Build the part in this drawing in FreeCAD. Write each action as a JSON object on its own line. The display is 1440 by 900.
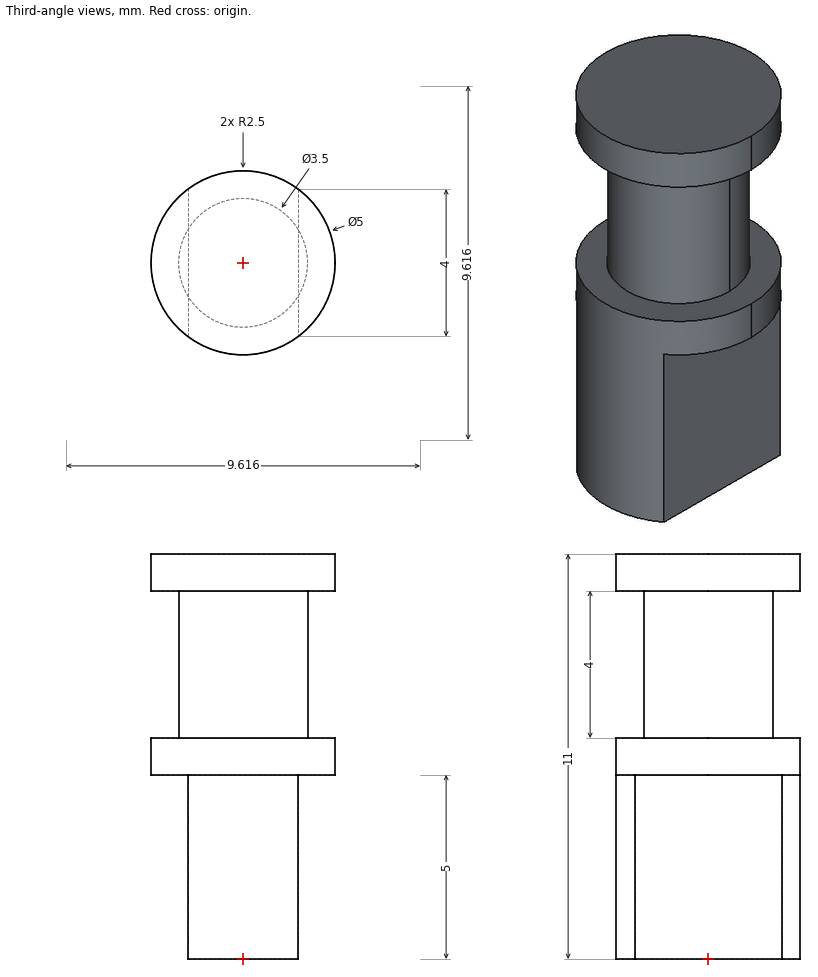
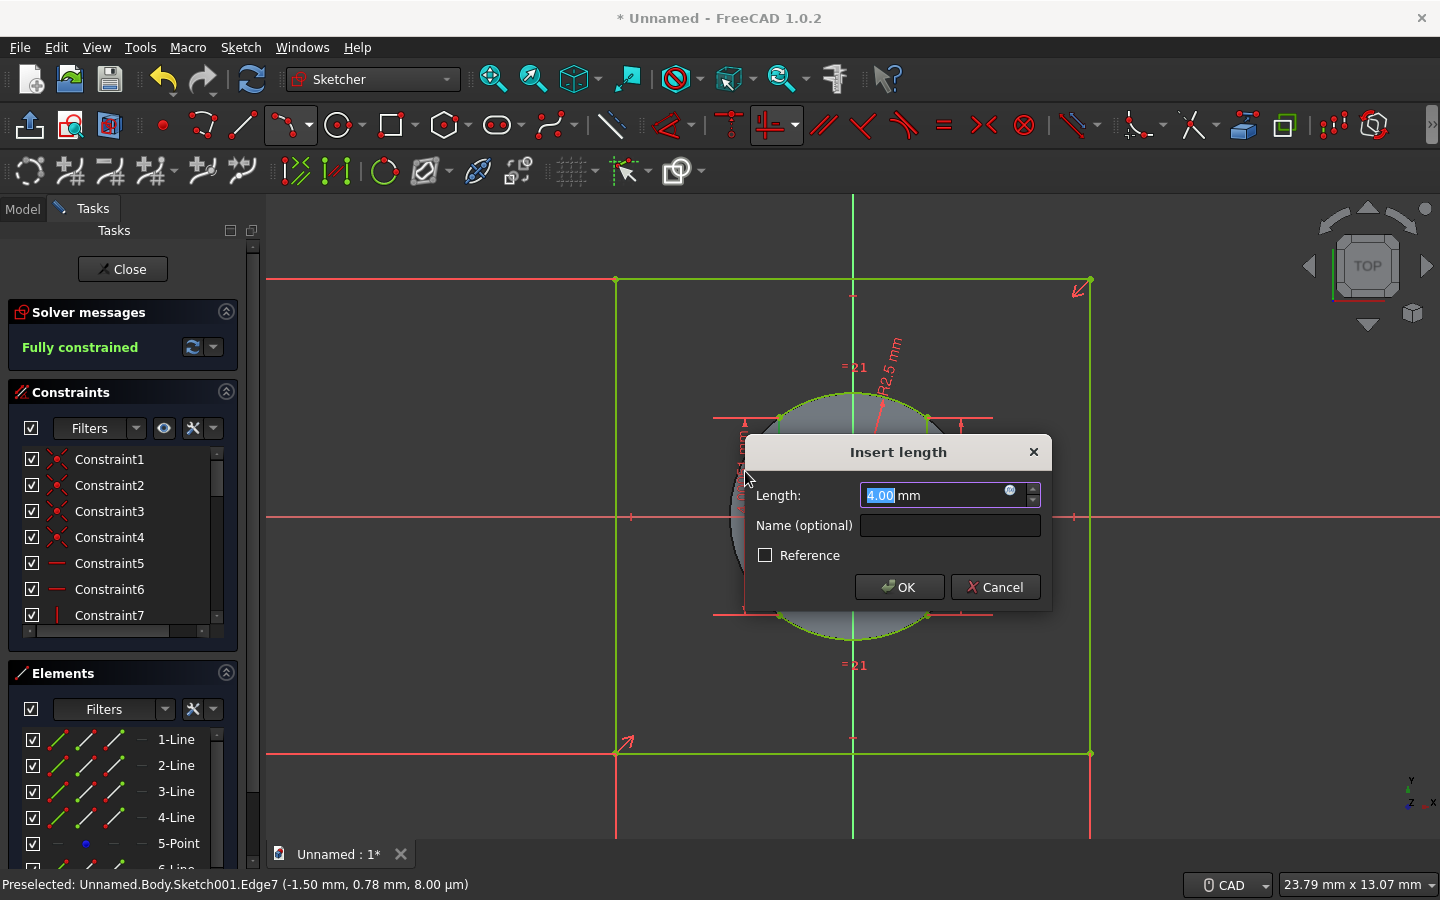
{"action": "type", "text": "4"}
{"action": "key", "text": "Return"}
{"action": "key", "text": "Escape"}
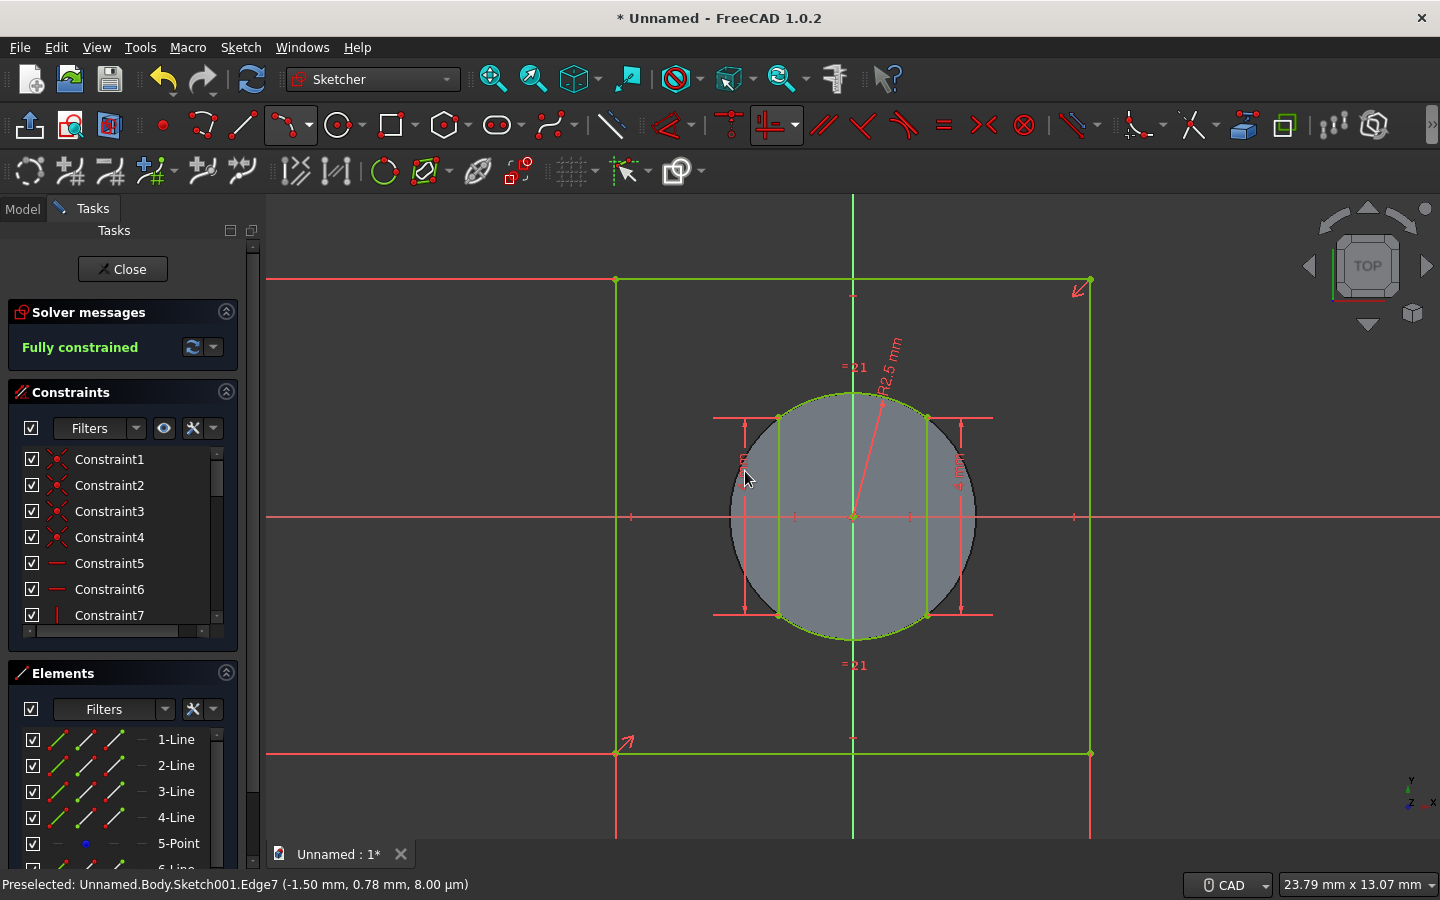
{"action": "left_click", "coordinate": [123, 269]}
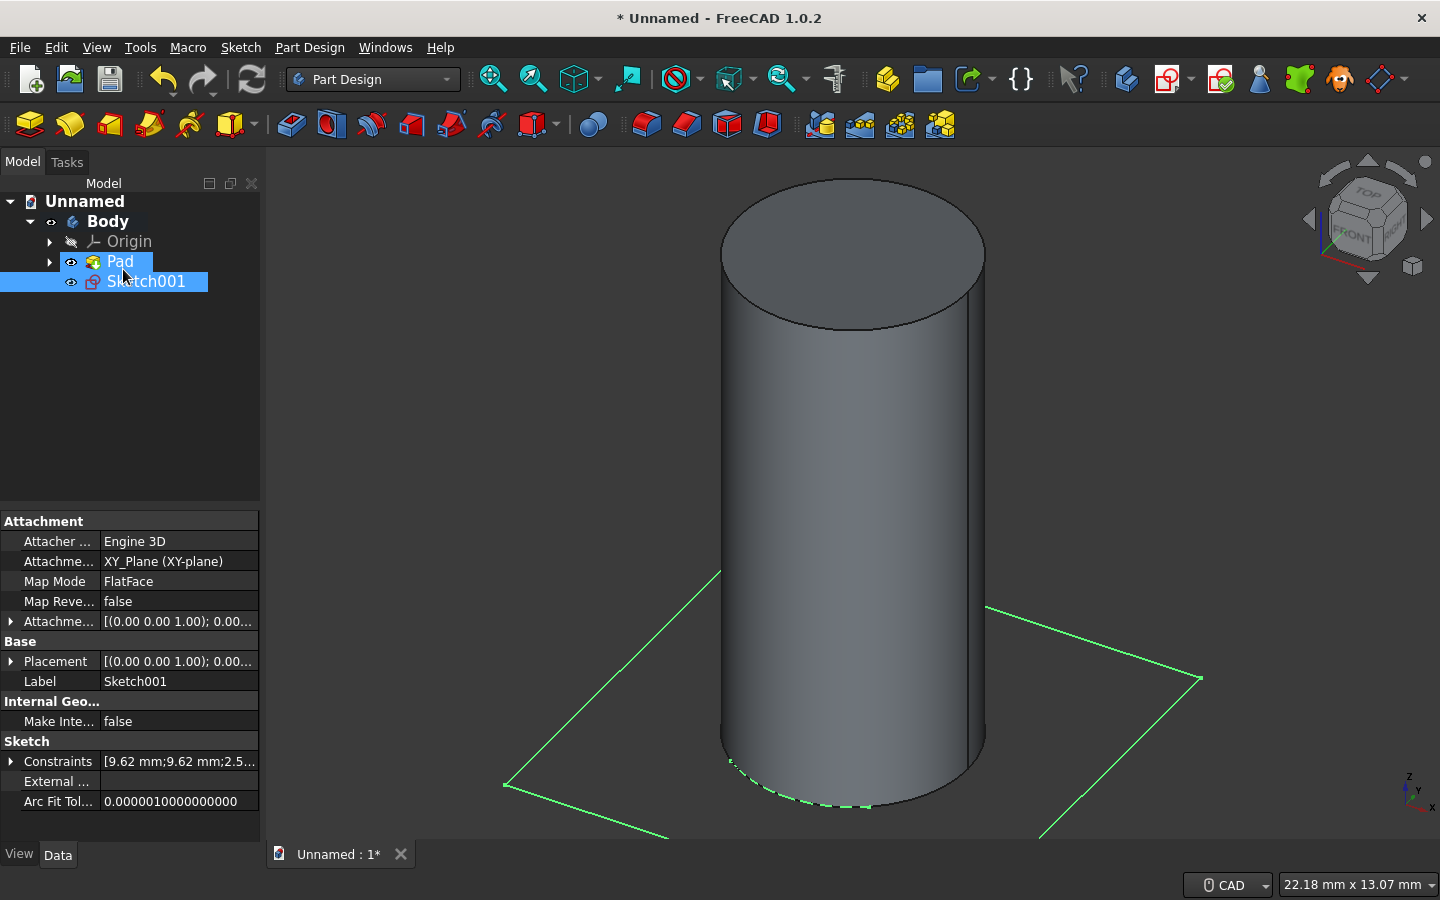
{"action": "left_click", "coordinate": [292, 124]}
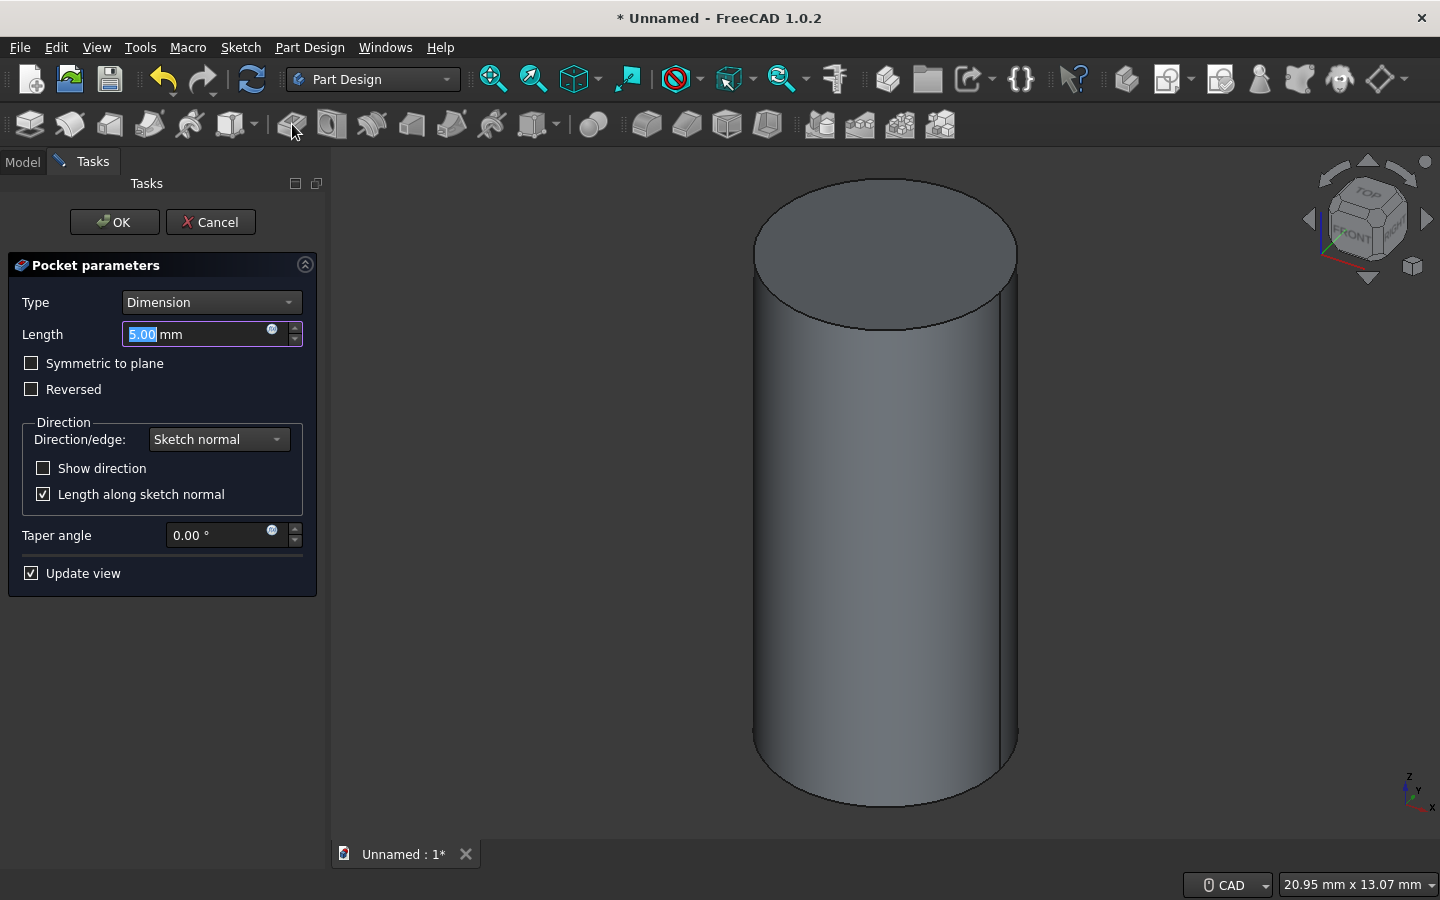
{"action": "type", "text": "5"}
{"action": "key", "text": "Tab"}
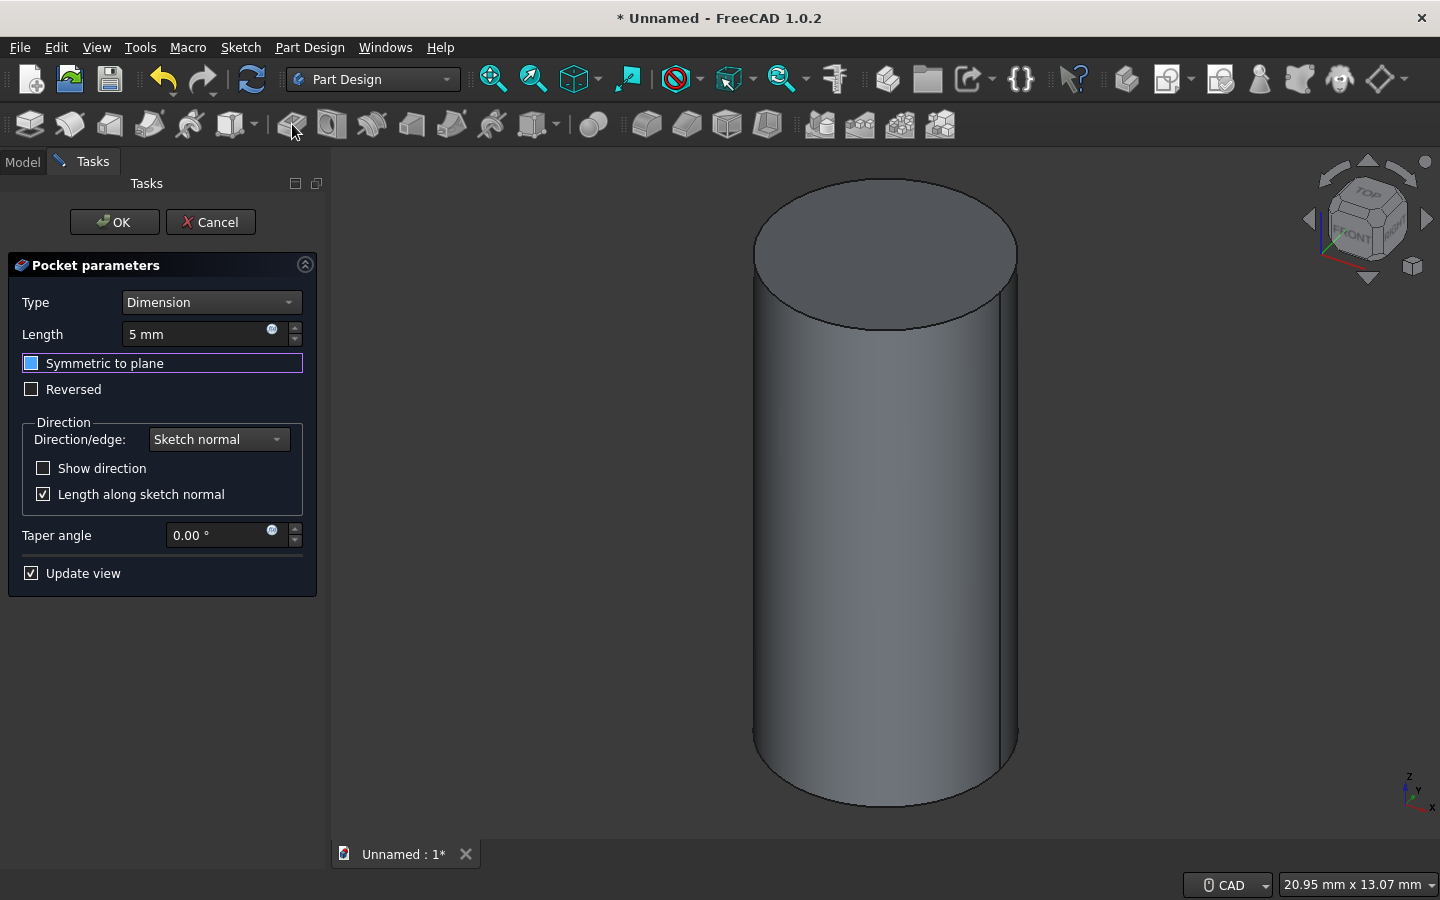
{"action": "left_click", "coordinate": [30, 389]}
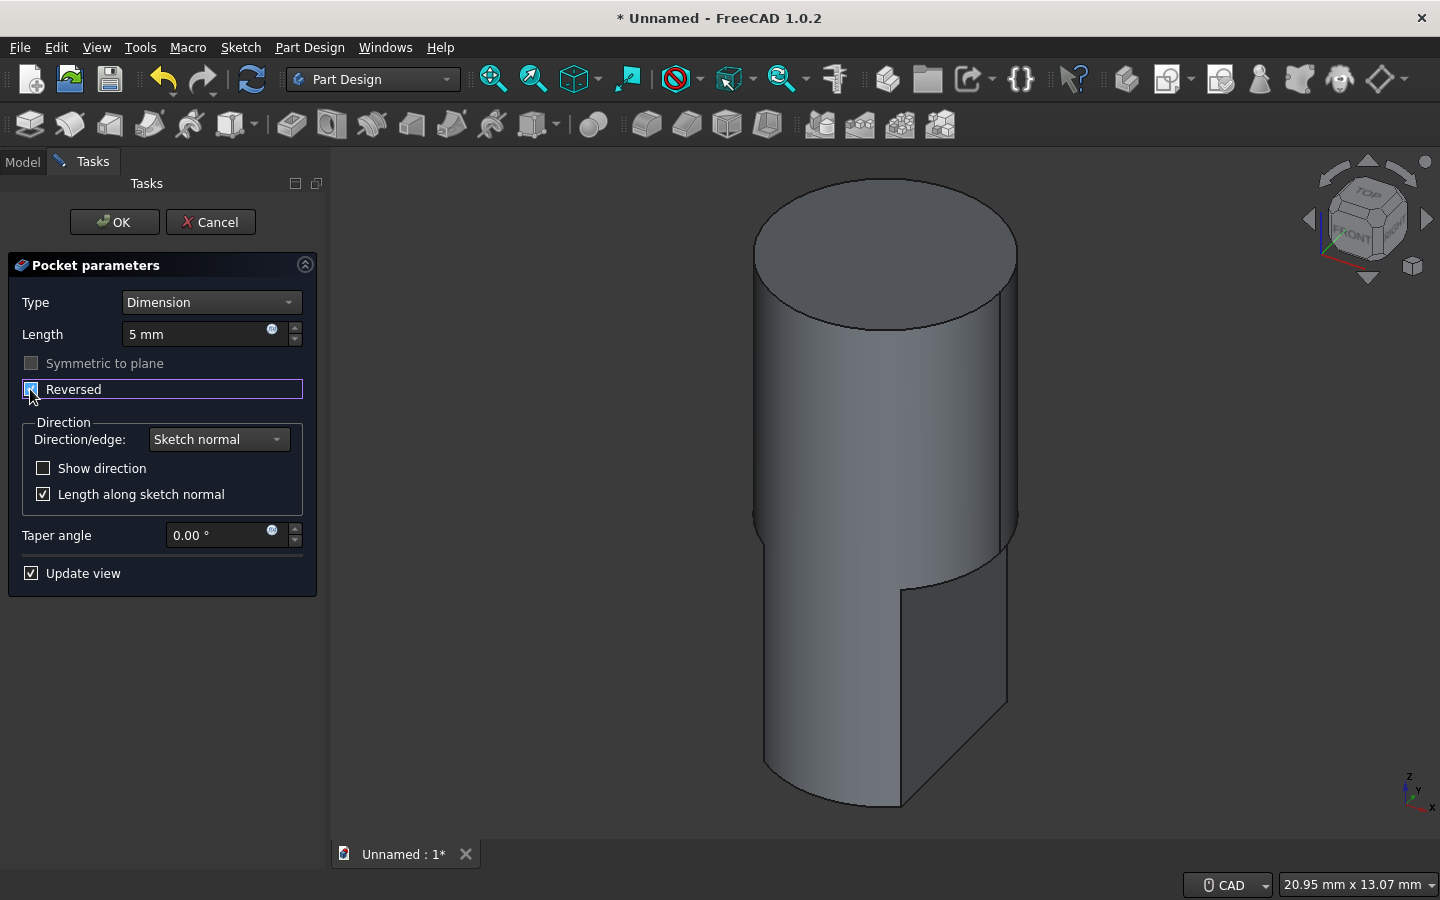
{"action": "left_click", "coordinate": [115, 222]}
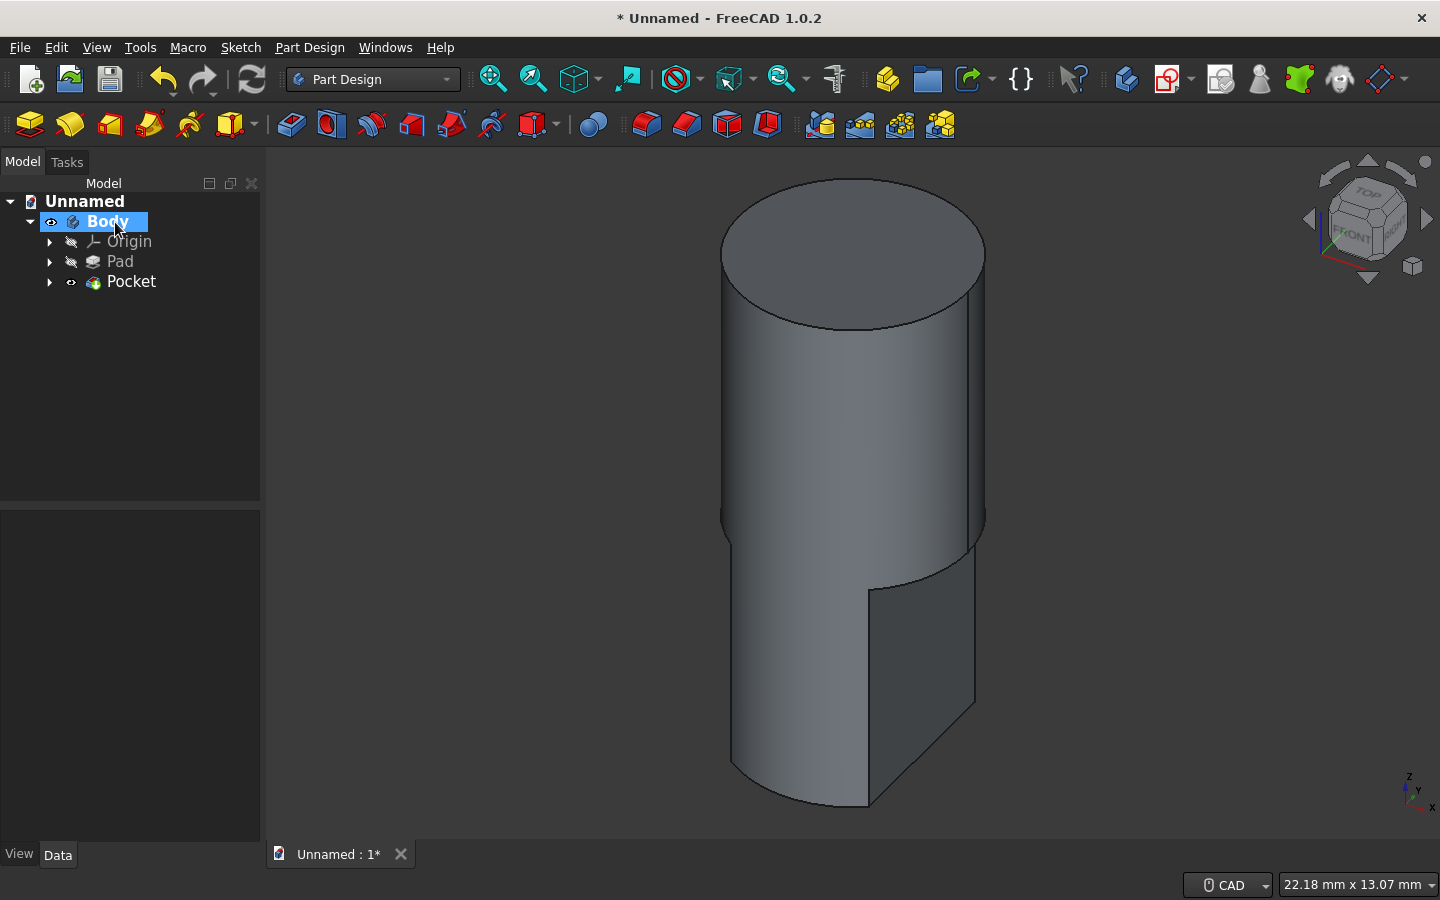
{"action": "left_click", "coordinate": [50, 242]}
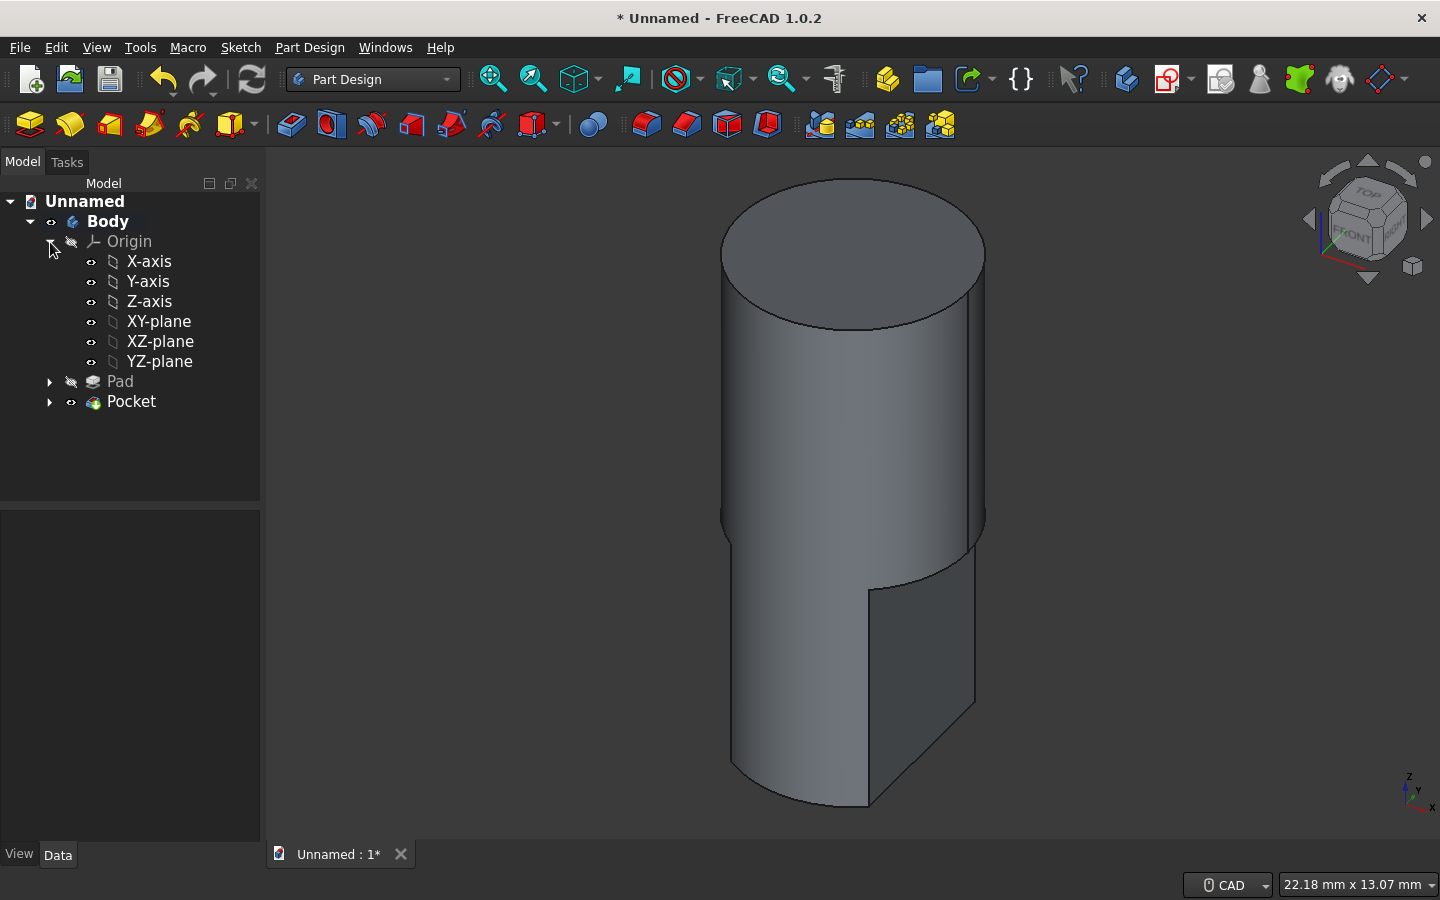
{"action": "left_click", "coordinate": [136, 322]}